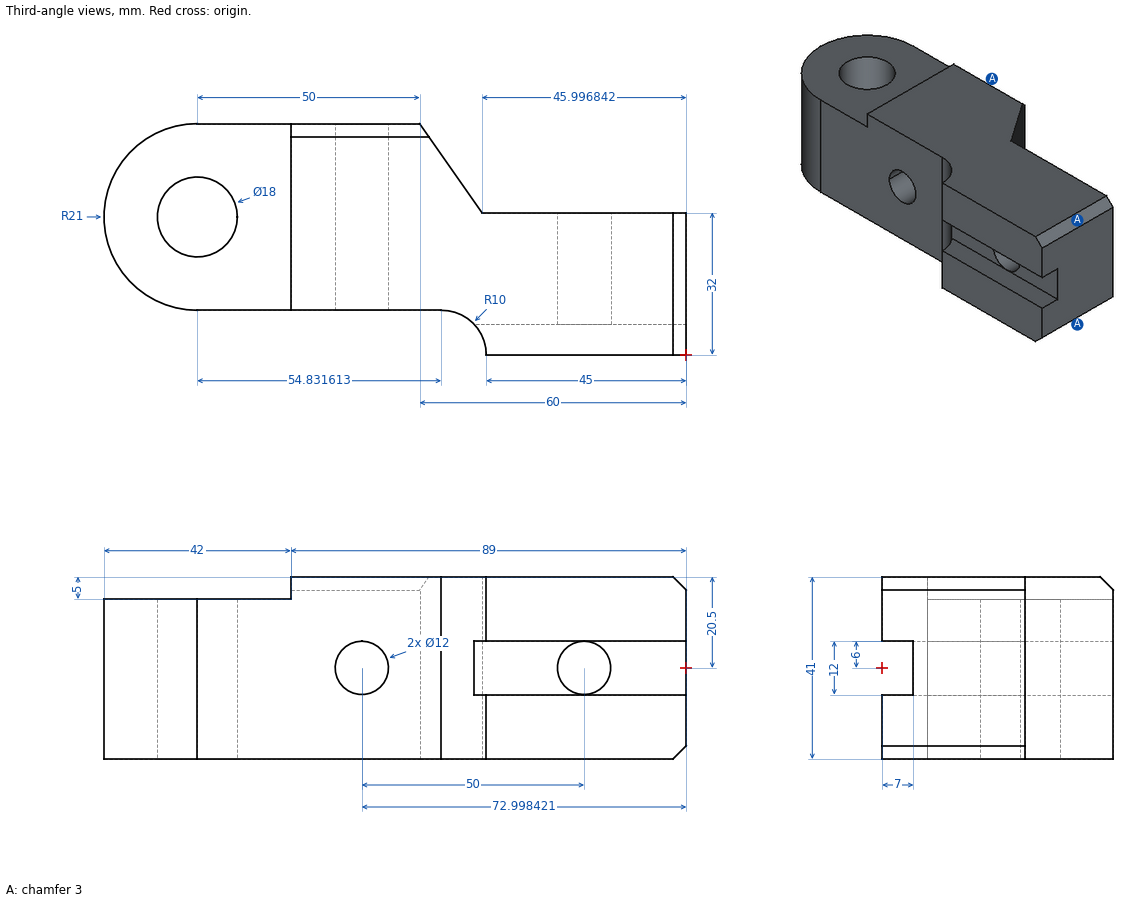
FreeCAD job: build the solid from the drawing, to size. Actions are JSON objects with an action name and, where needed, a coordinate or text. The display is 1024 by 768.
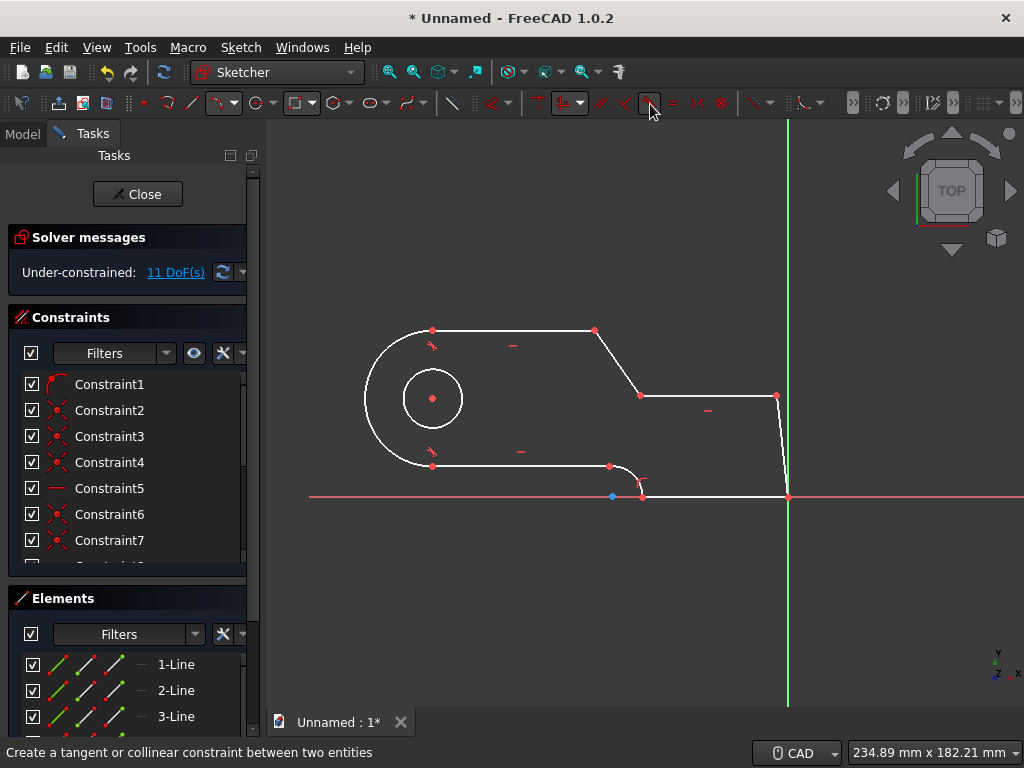
{"action": "left_click", "coordinate": [785, 467]}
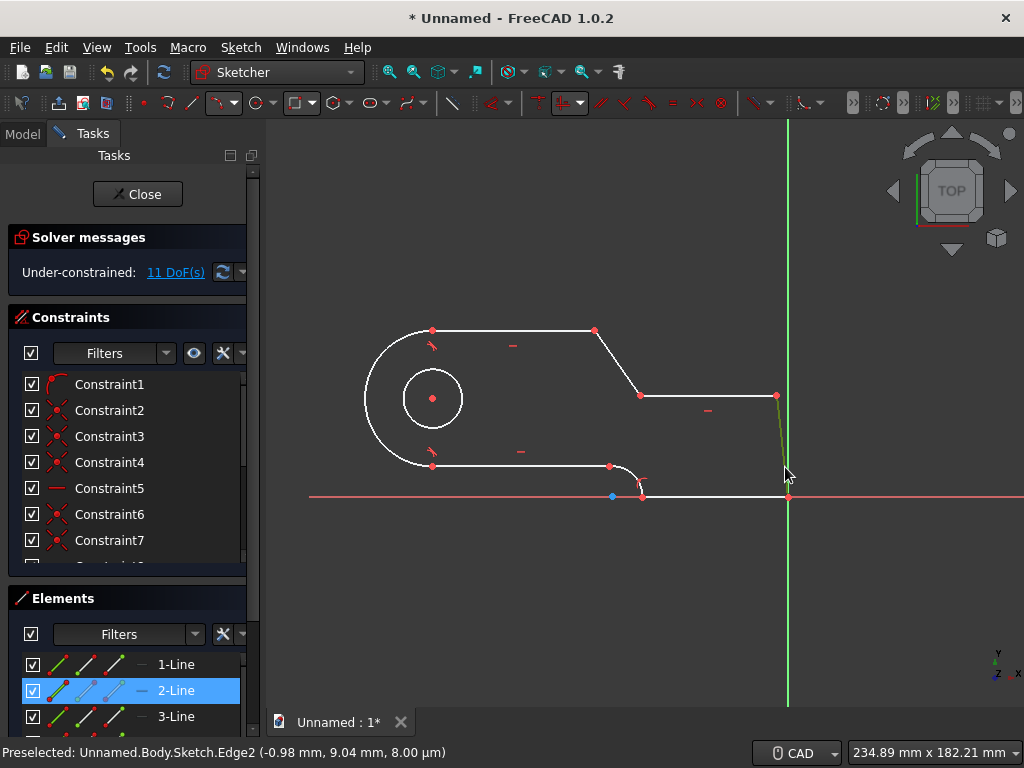
{"action": "left_click", "coordinate": [582, 104]}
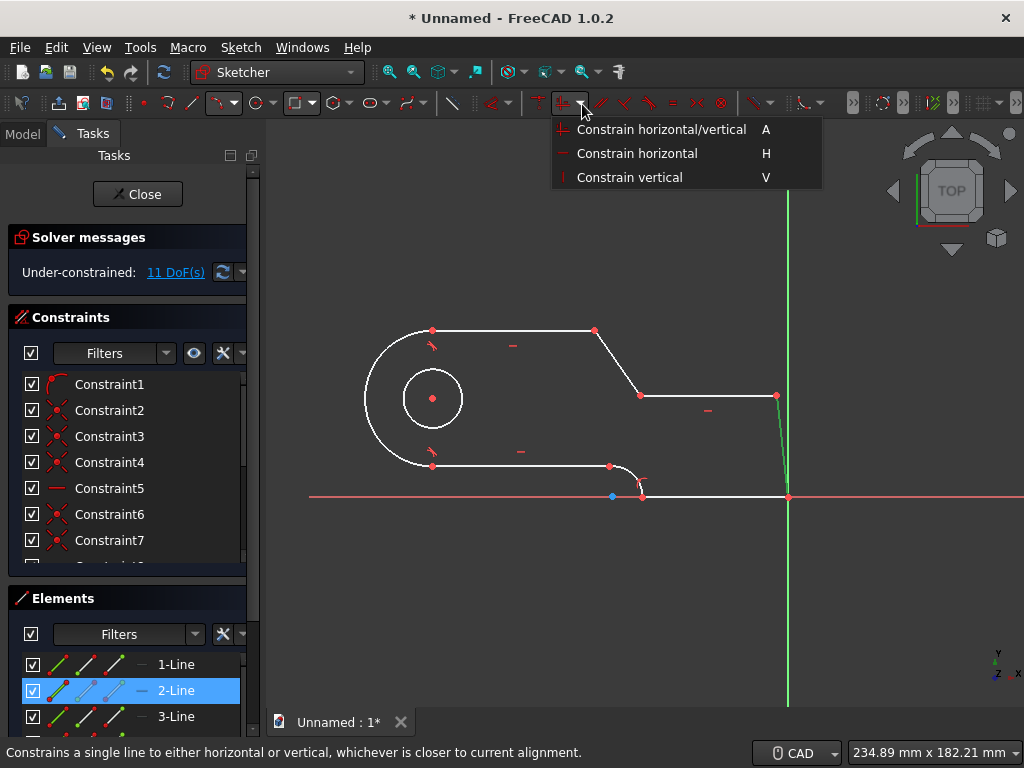
{"action": "left_click", "coordinate": [687, 177]}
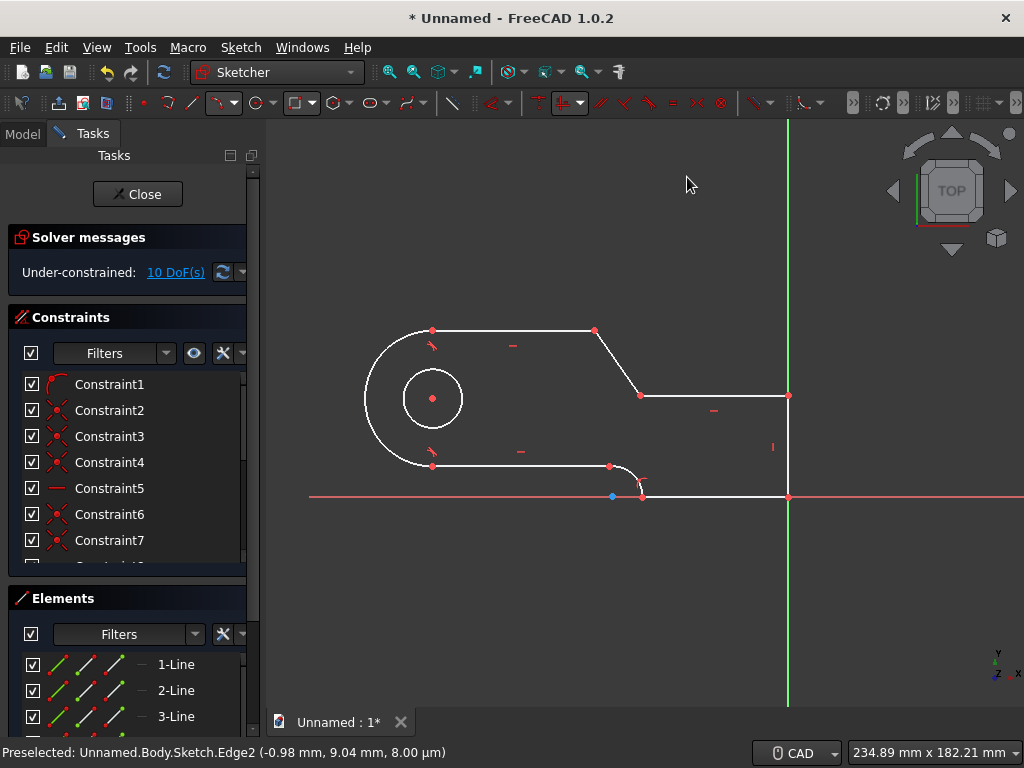
{"action": "left_click", "coordinate": [612, 497]}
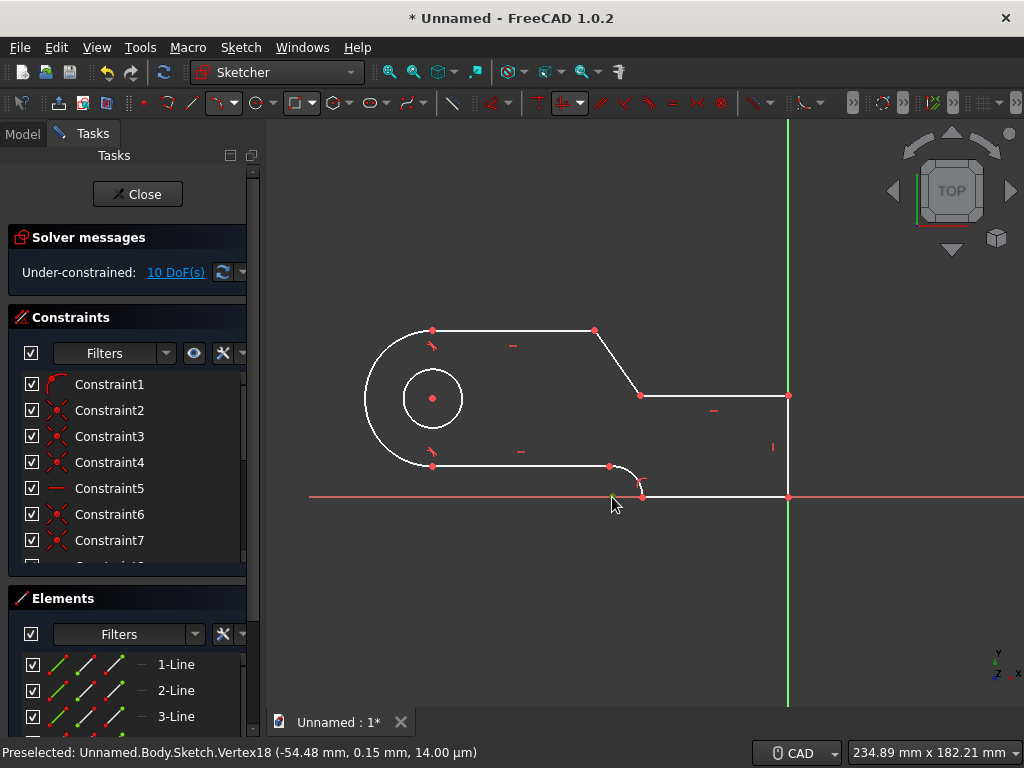
{"action": "left_click", "coordinate": [334, 497]}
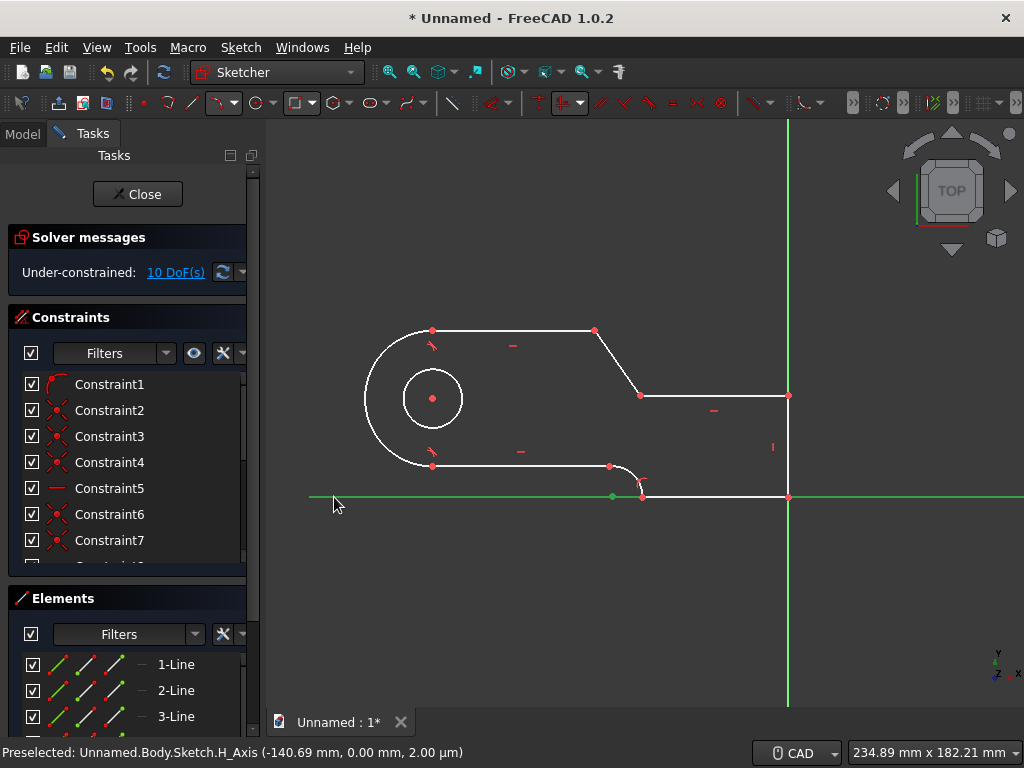
{"action": "left_click", "coordinate": [538, 104]}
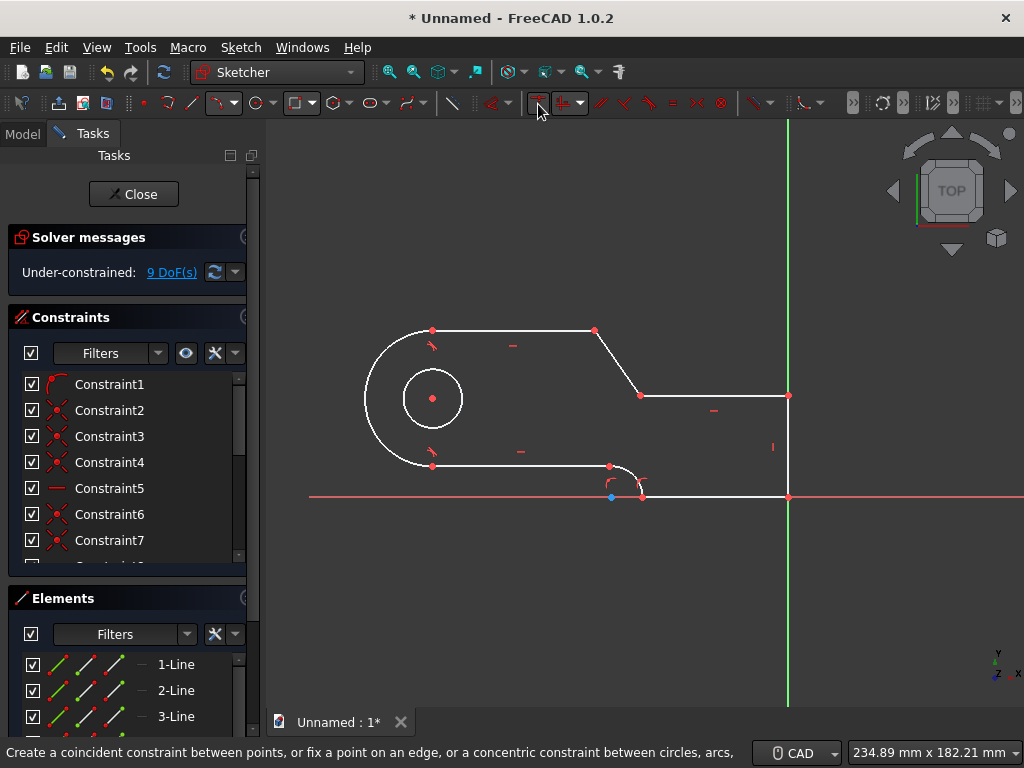
{"action": "left_click", "coordinate": [492, 104]}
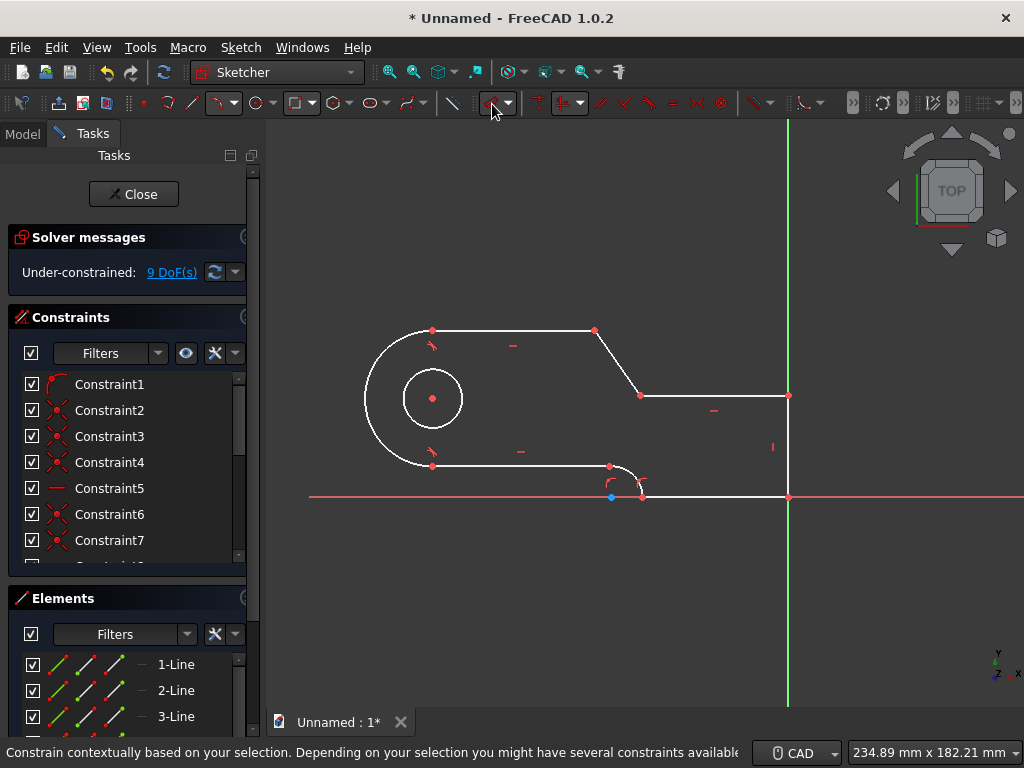
{"action": "left_click", "coordinate": [378, 359]}
{"action": "left_click", "coordinate": [352, 340]}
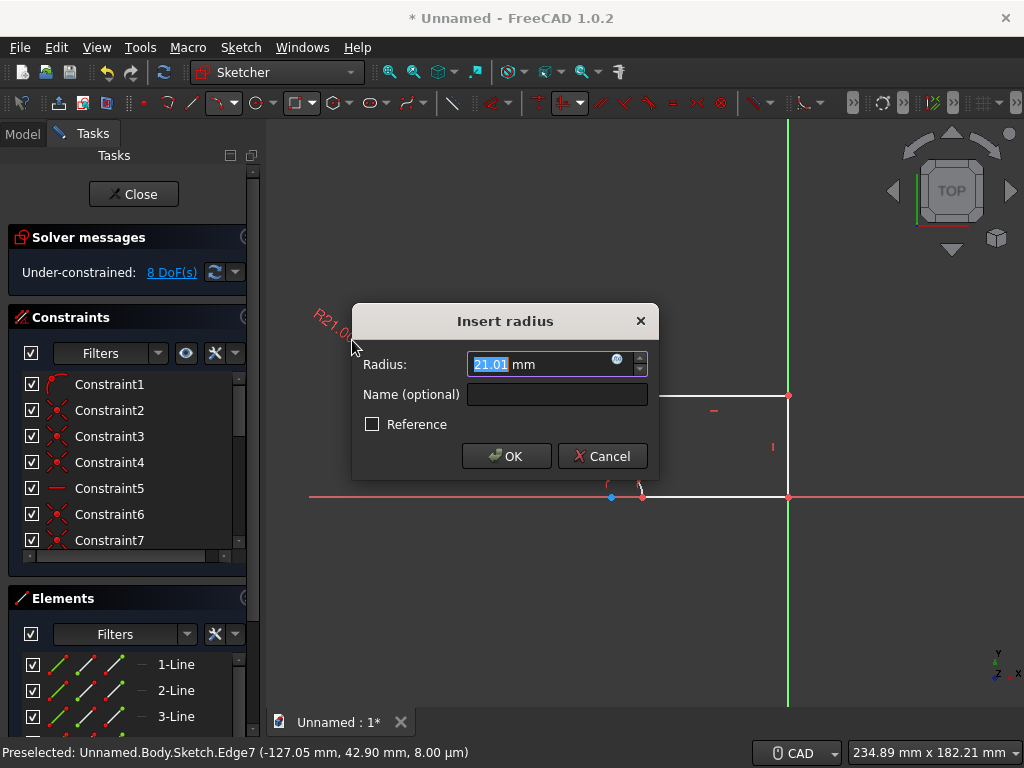
{"action": "type", "text": "21"}
{"action": "key", "text": "Return"}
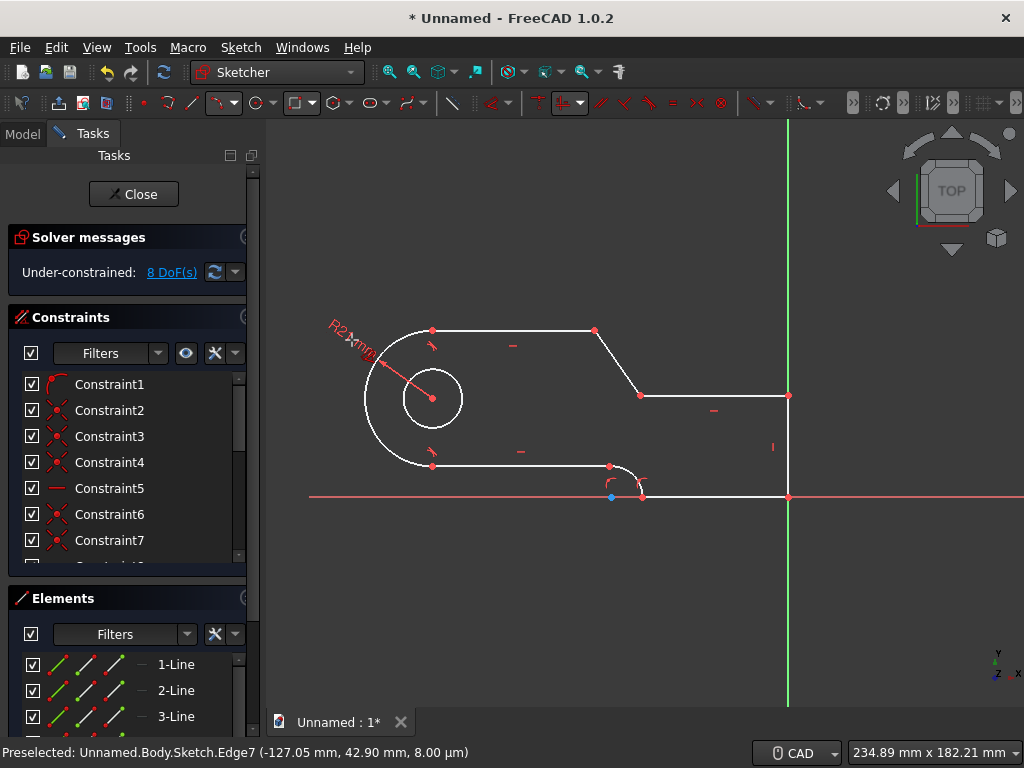
{"action": "scroll", "coordinate": [639, 483], "scroll_direction": "up", "scroll_amount": 2}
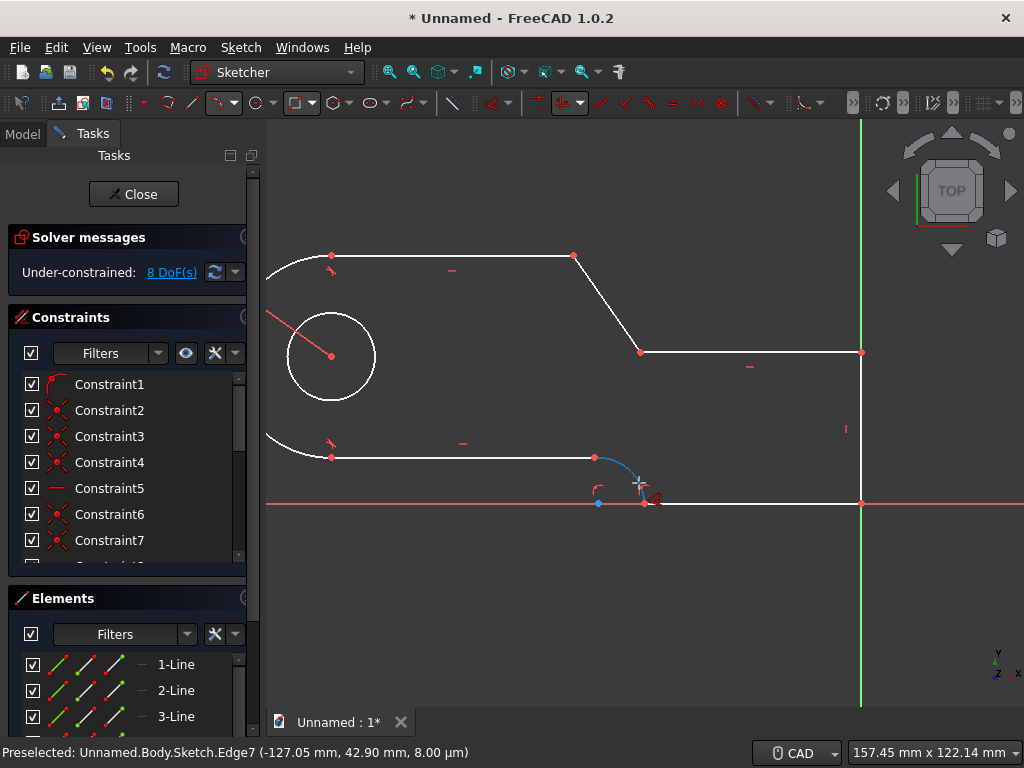
{"action": "left_click", "coordinate": [639, 482]}
{"action": "left_click", "coordinate": [667, 467]}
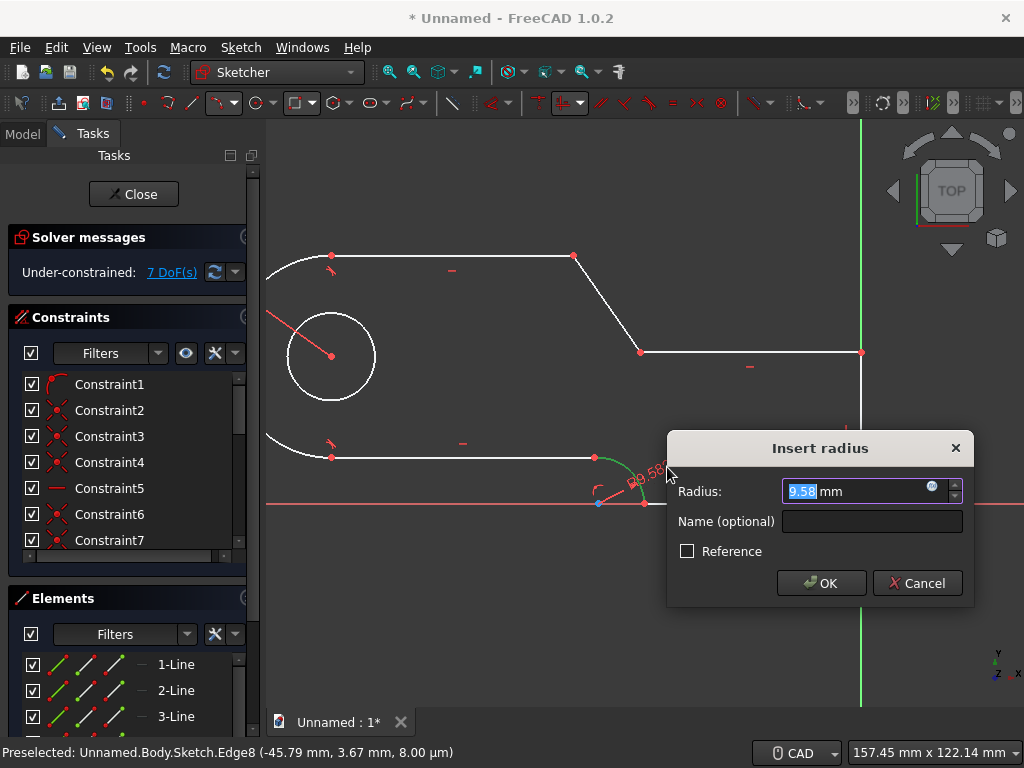
{"action": "type", "text": "10"}
{"action": "key", "text": "Return"}